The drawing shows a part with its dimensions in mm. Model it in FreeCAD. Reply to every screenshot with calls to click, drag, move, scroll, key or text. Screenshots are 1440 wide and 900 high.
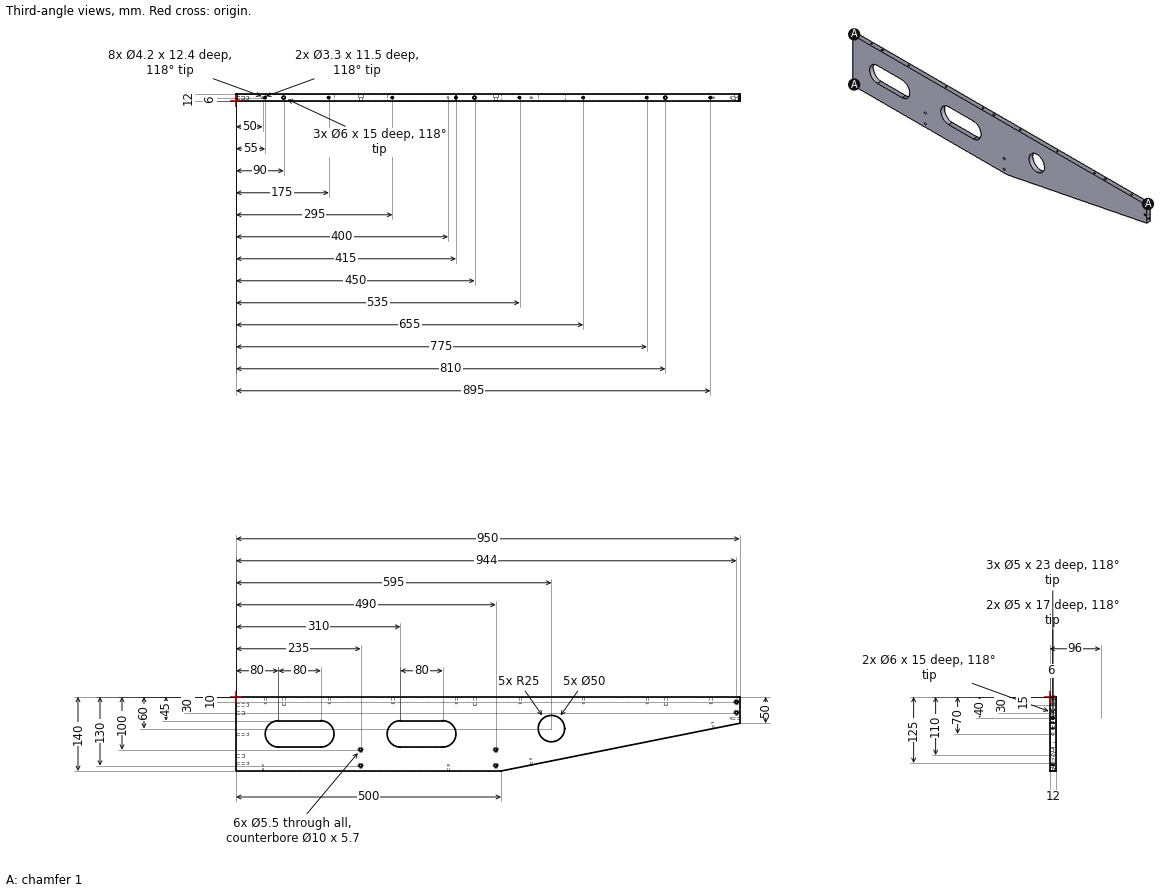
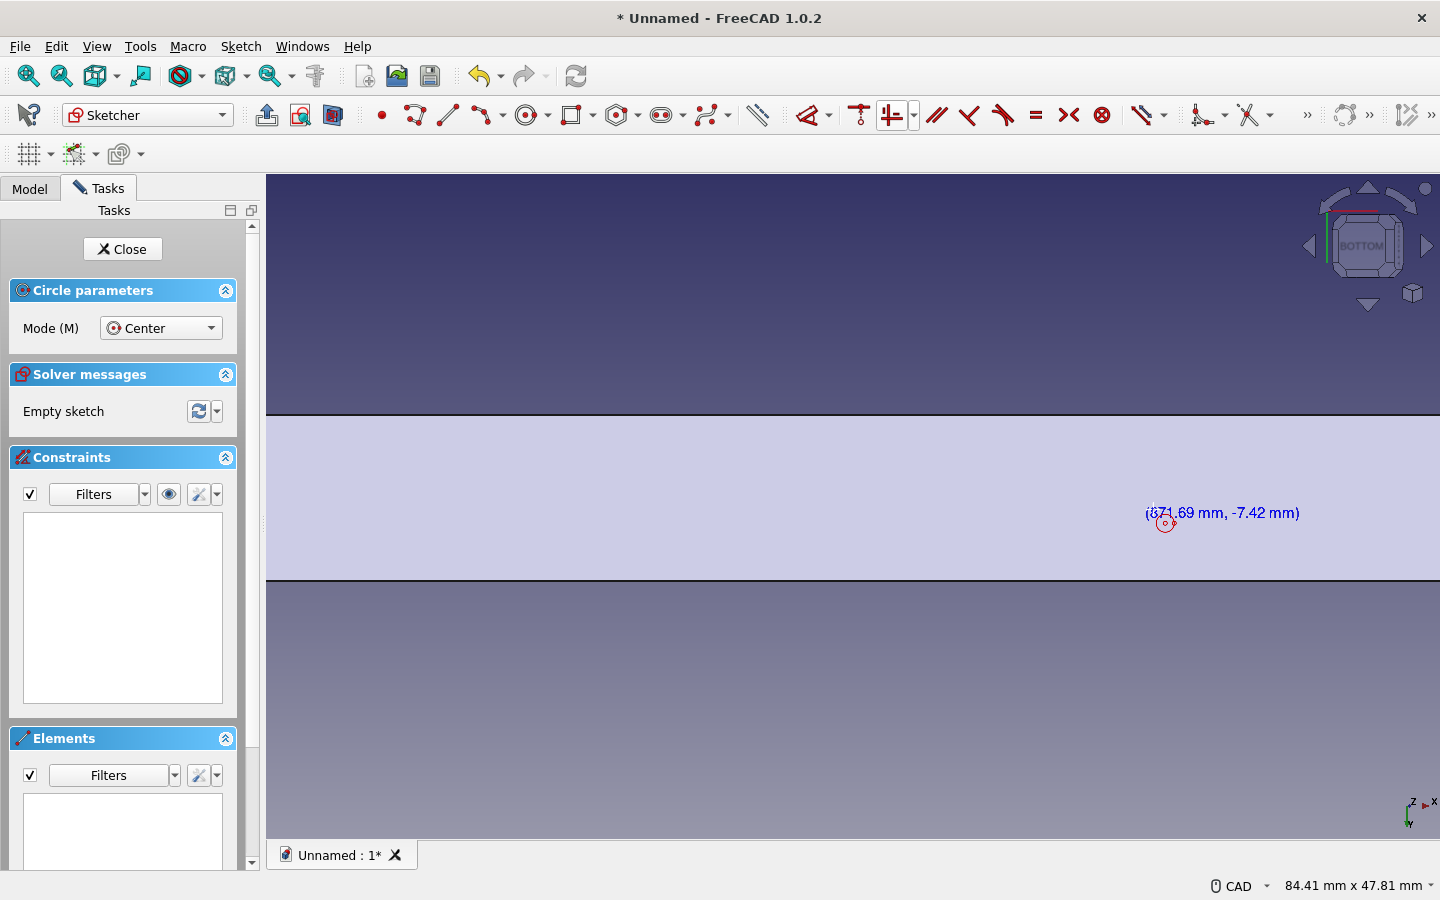
scroll(1153, 509, down, 14)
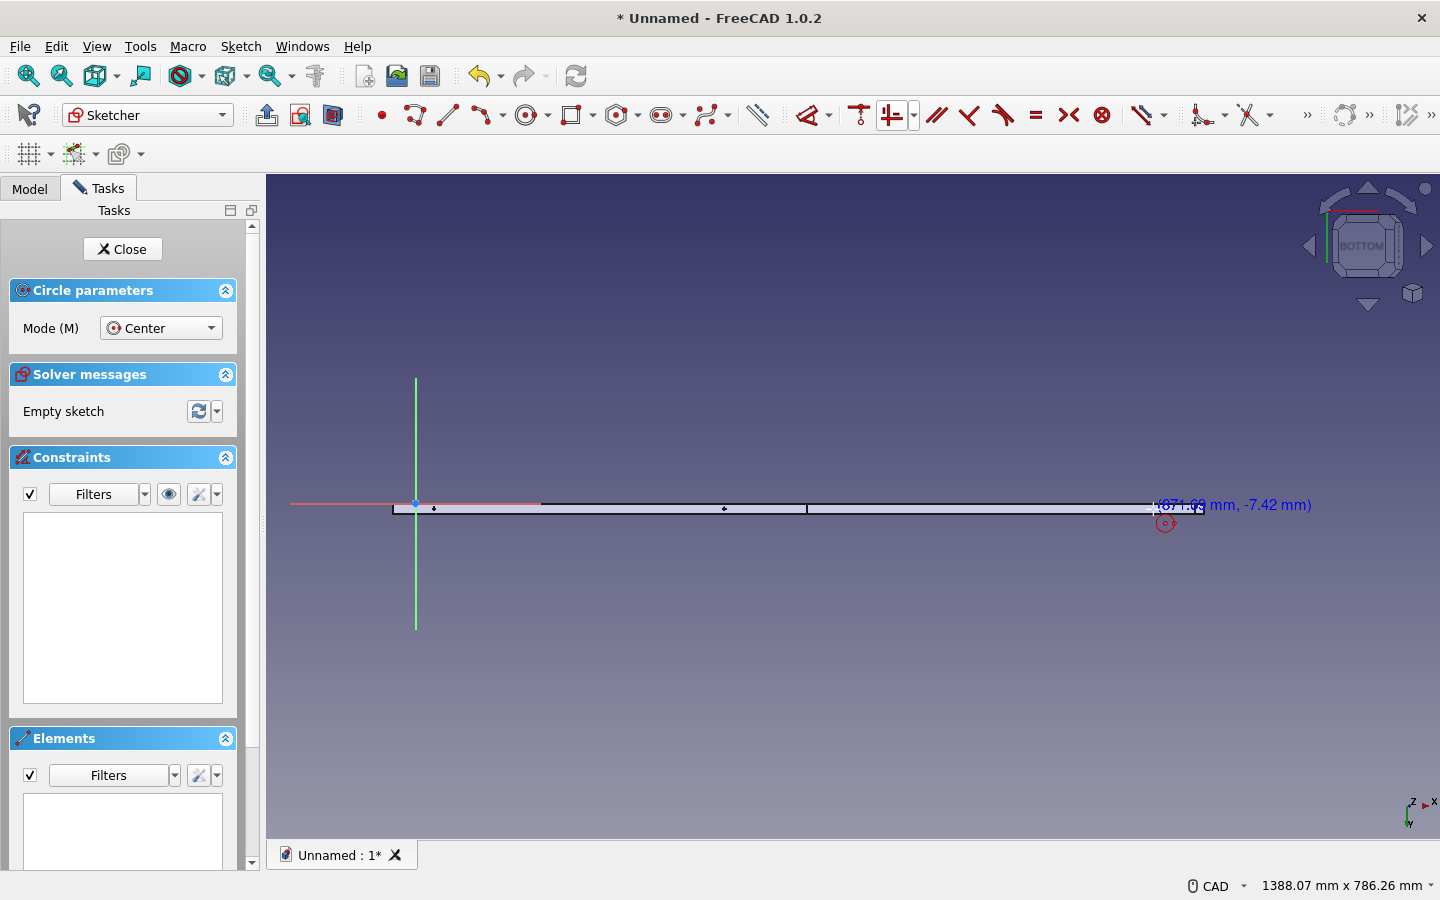
scroll(1153, 509, up, 6)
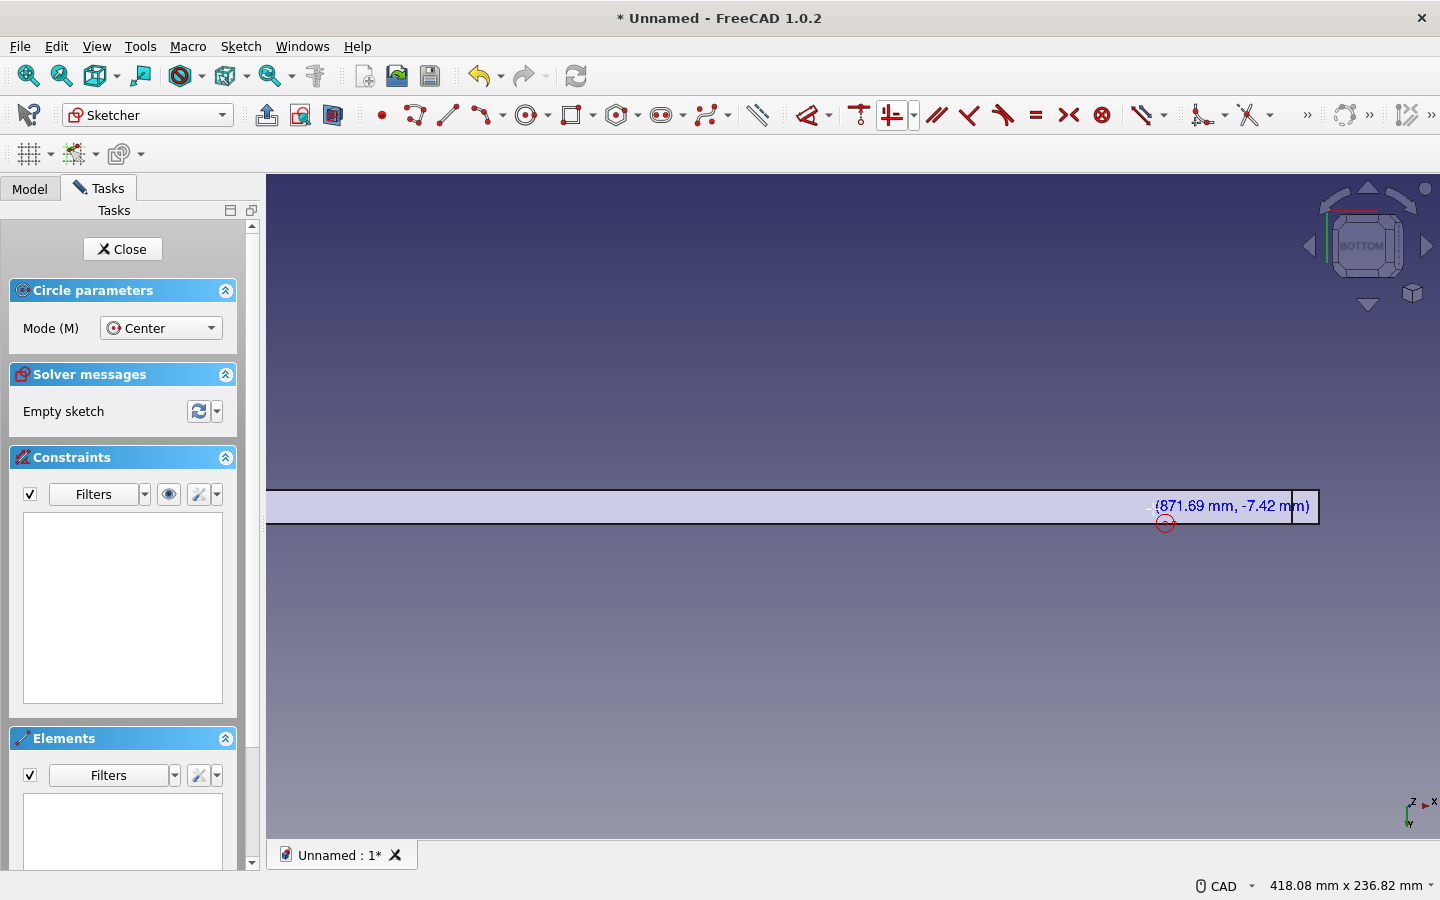
click(1151, 507)
move(1155, 510)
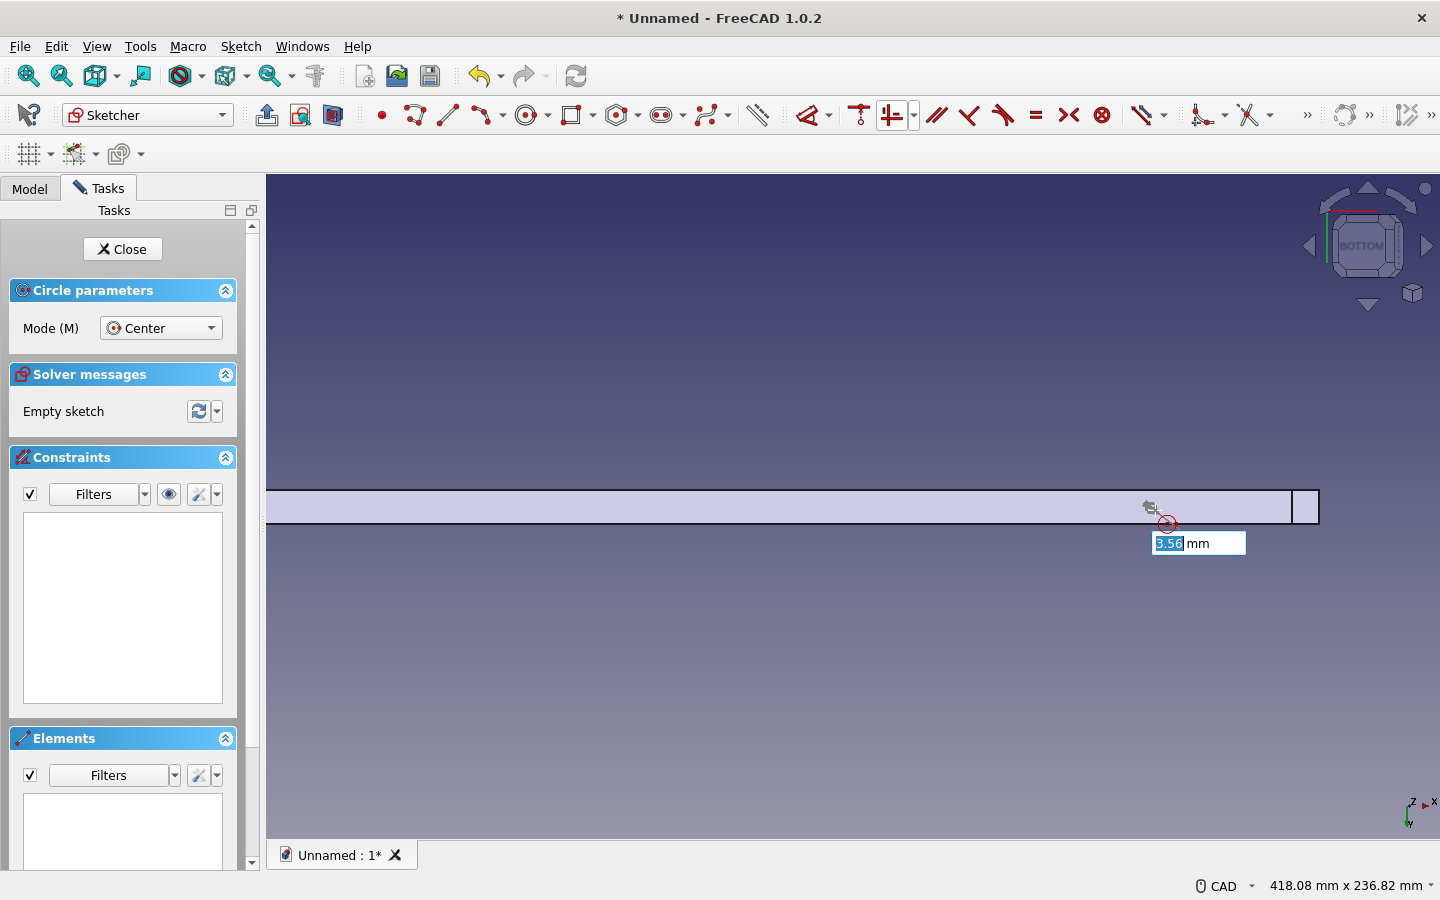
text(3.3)
key(Return)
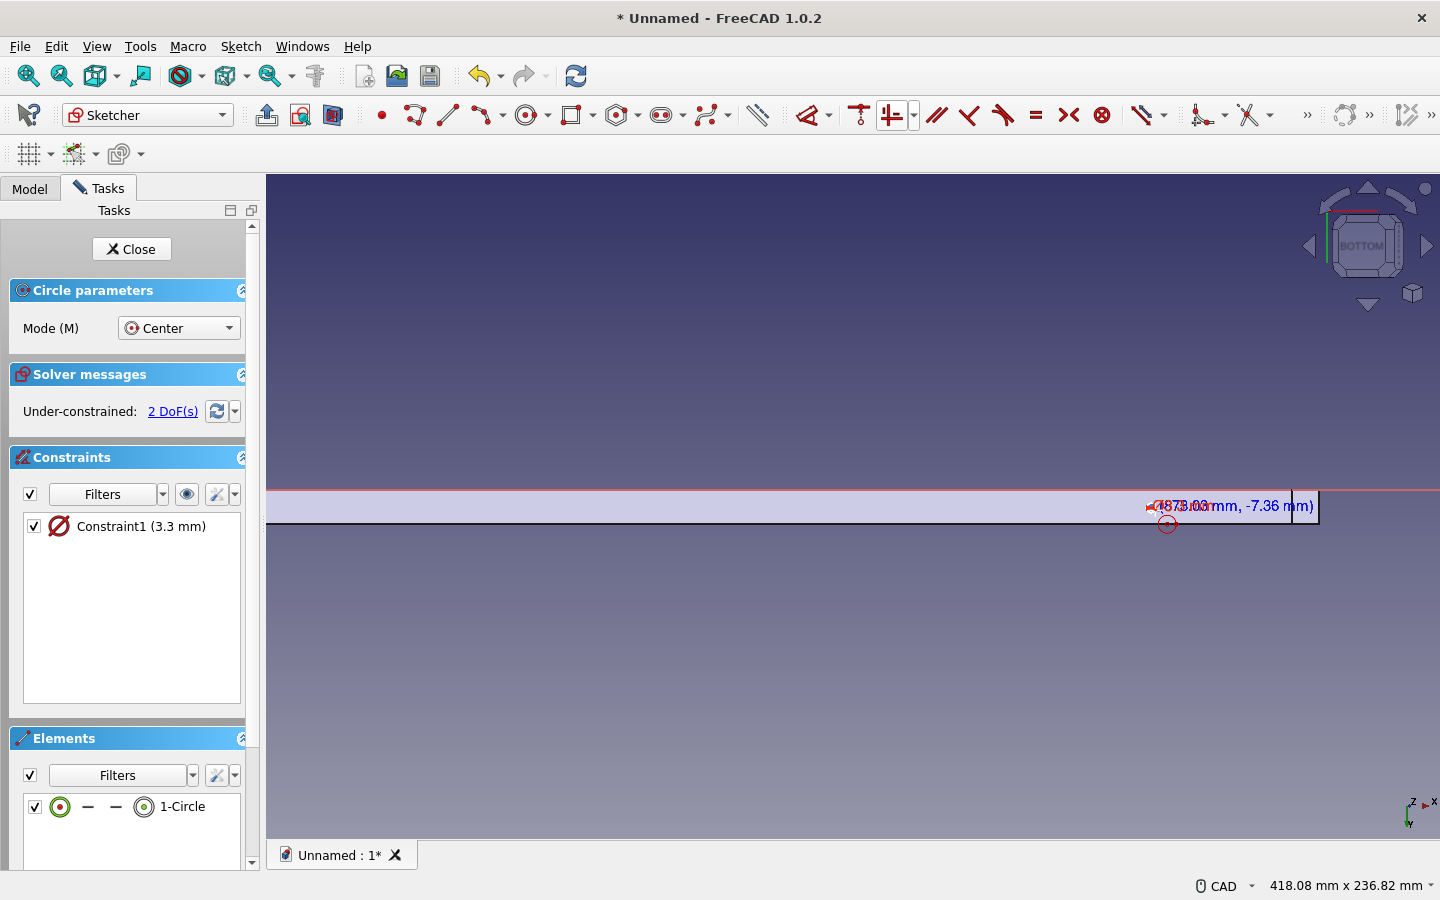
scroll(1153, 509, down, 6)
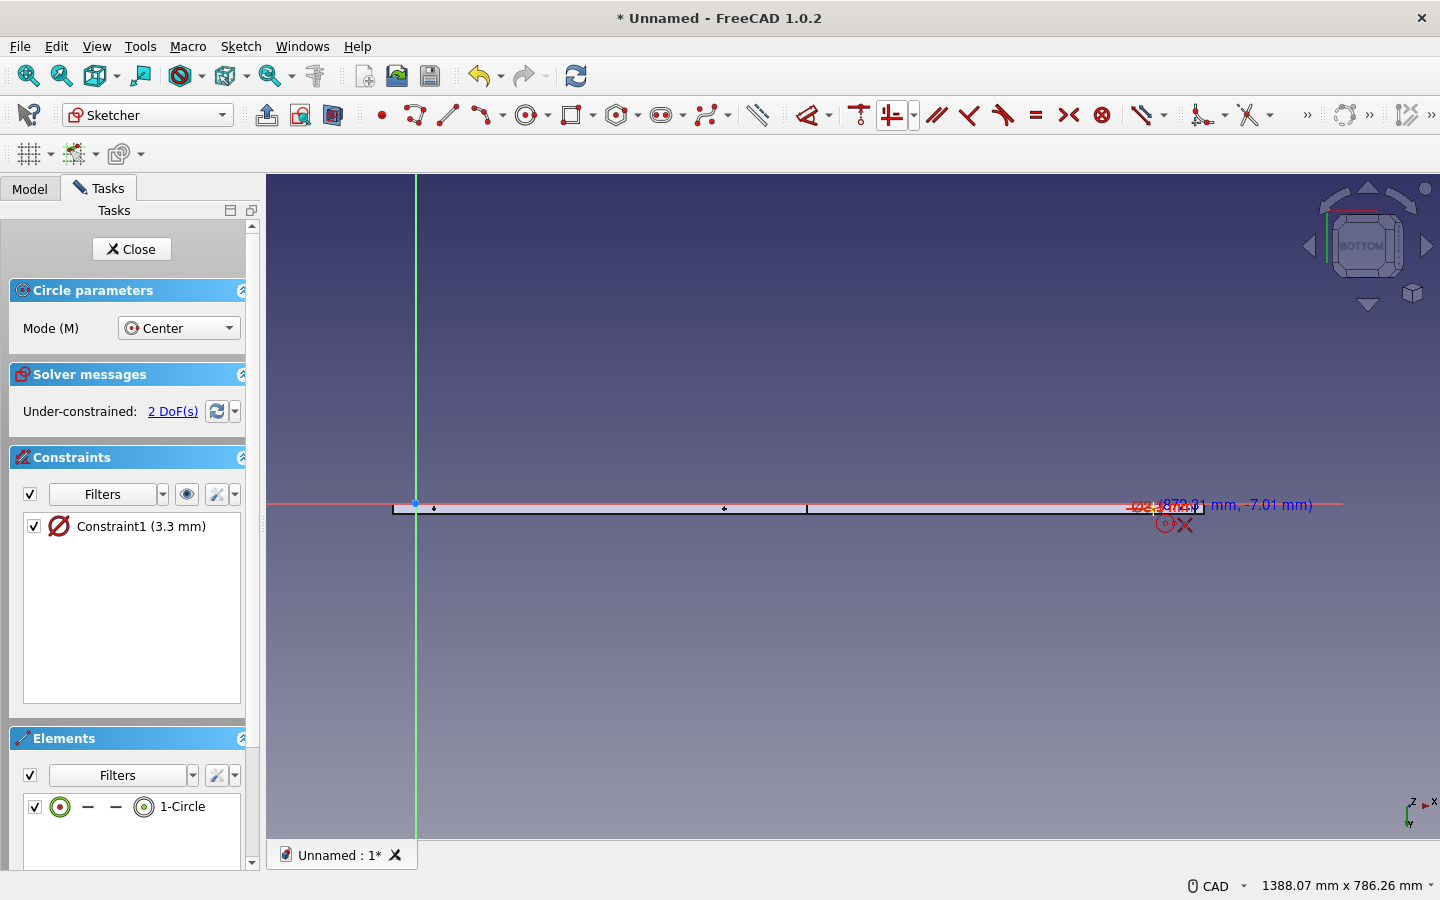
scroll(857, 509, up, 14)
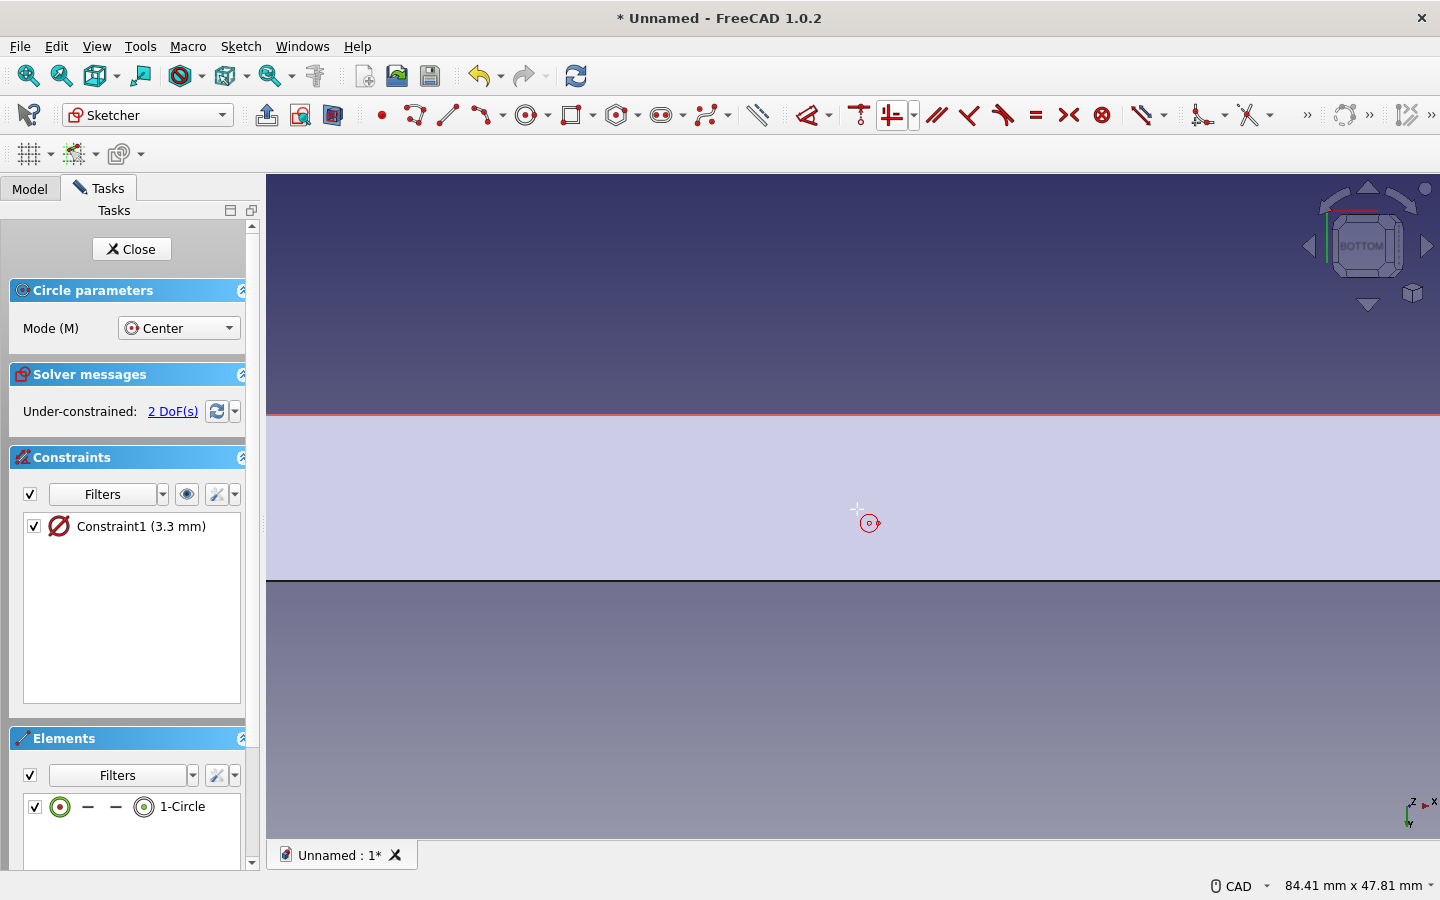
scroll(857, 509, down, 14)